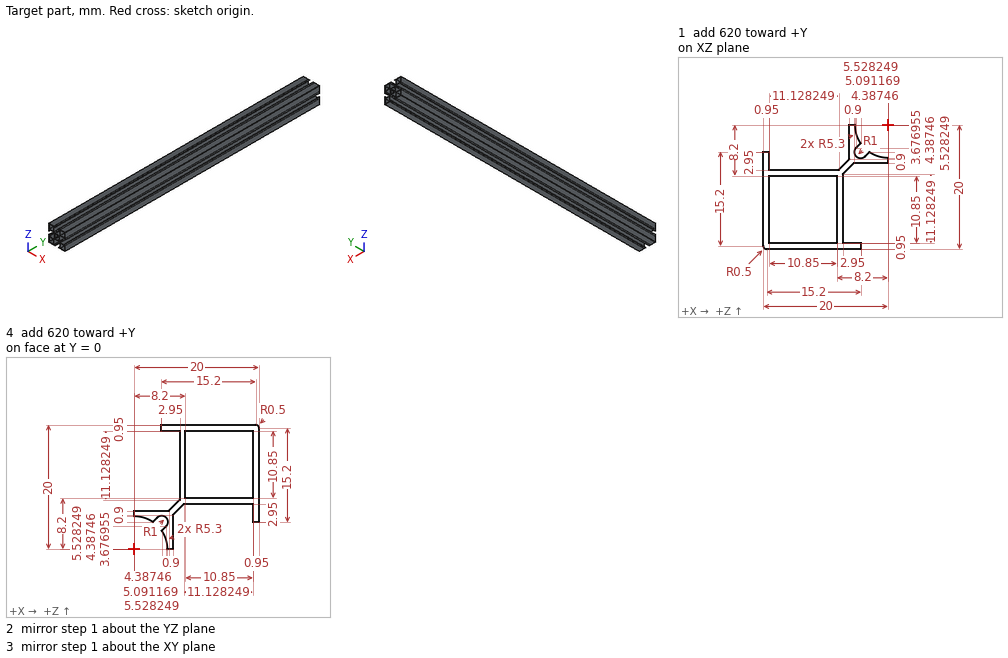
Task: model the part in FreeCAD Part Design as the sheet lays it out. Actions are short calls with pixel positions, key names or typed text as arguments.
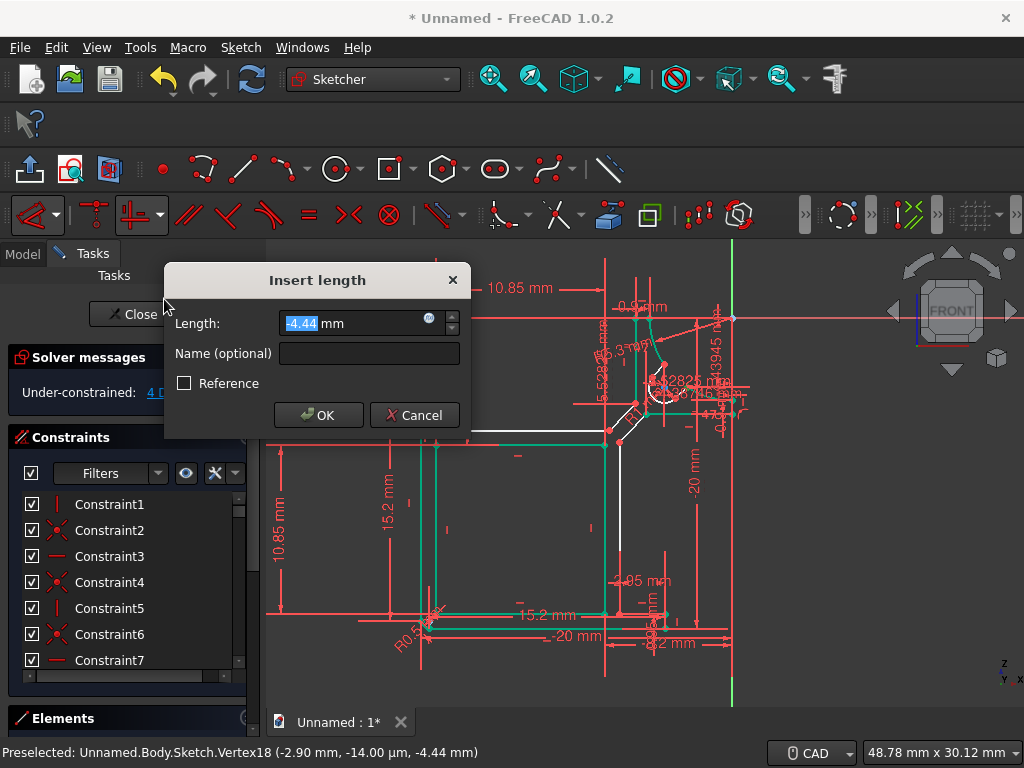
text(-4.38746)
key(Return)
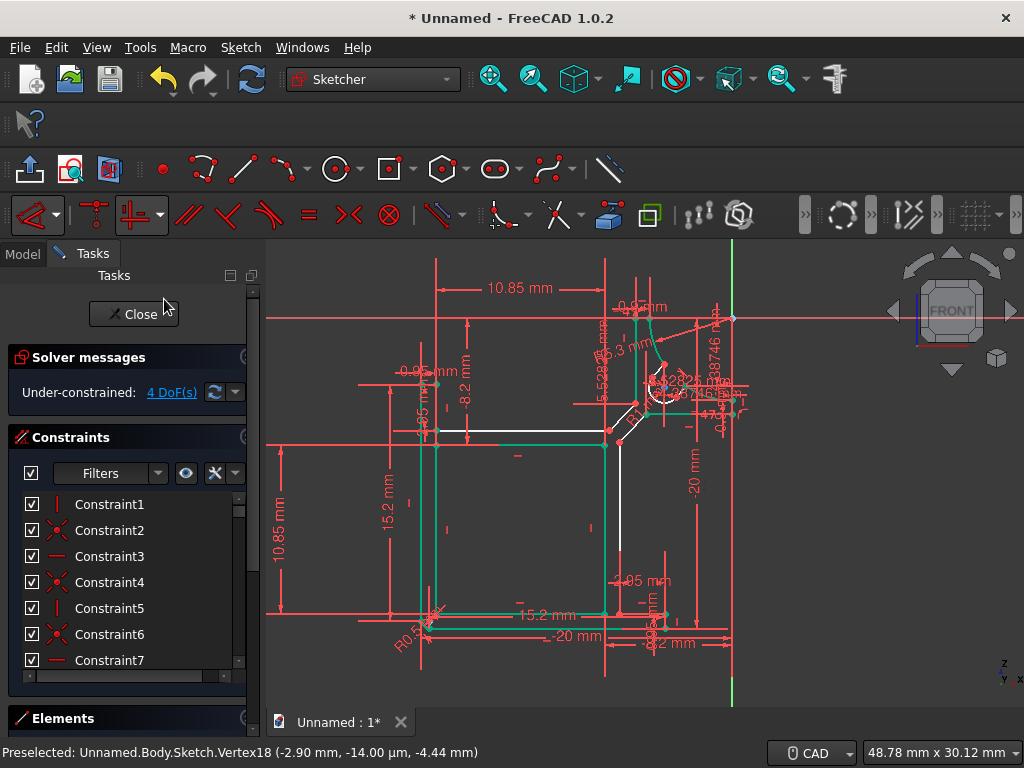
click(488, 431)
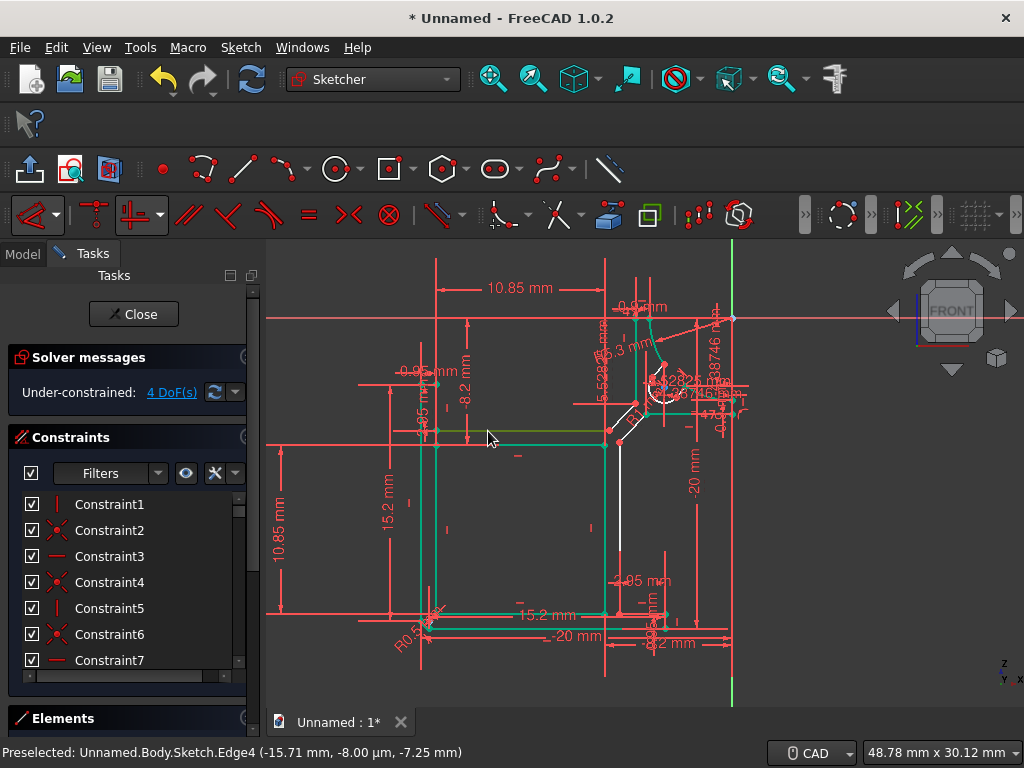
click(58, 216)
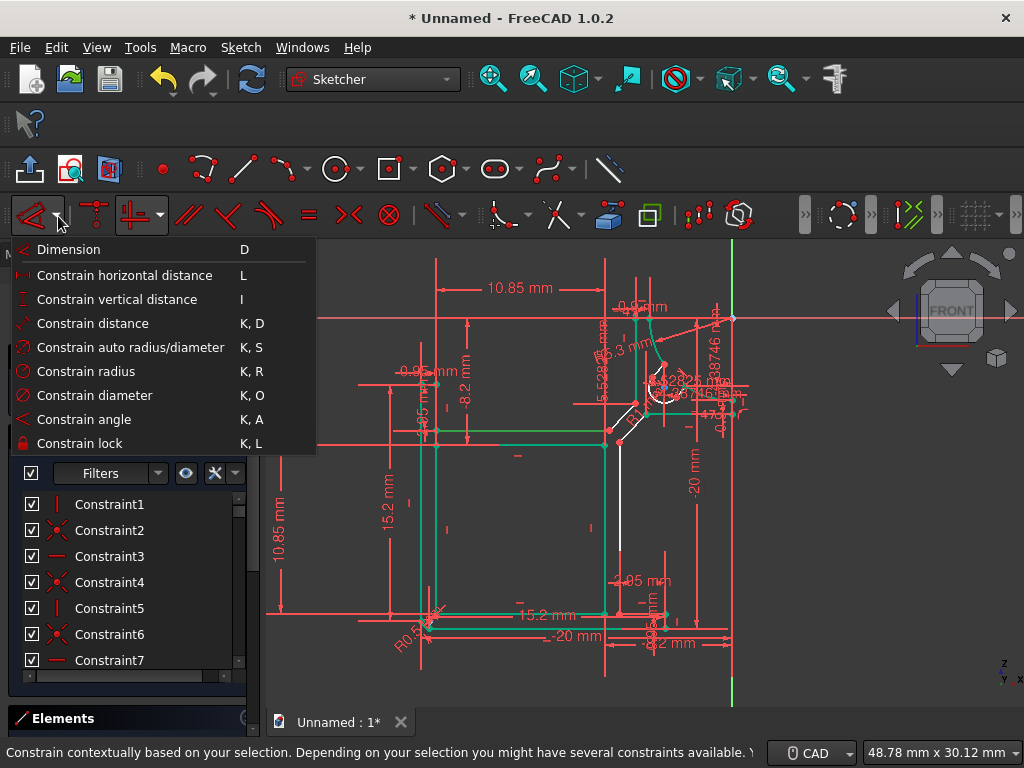
click(164, 275)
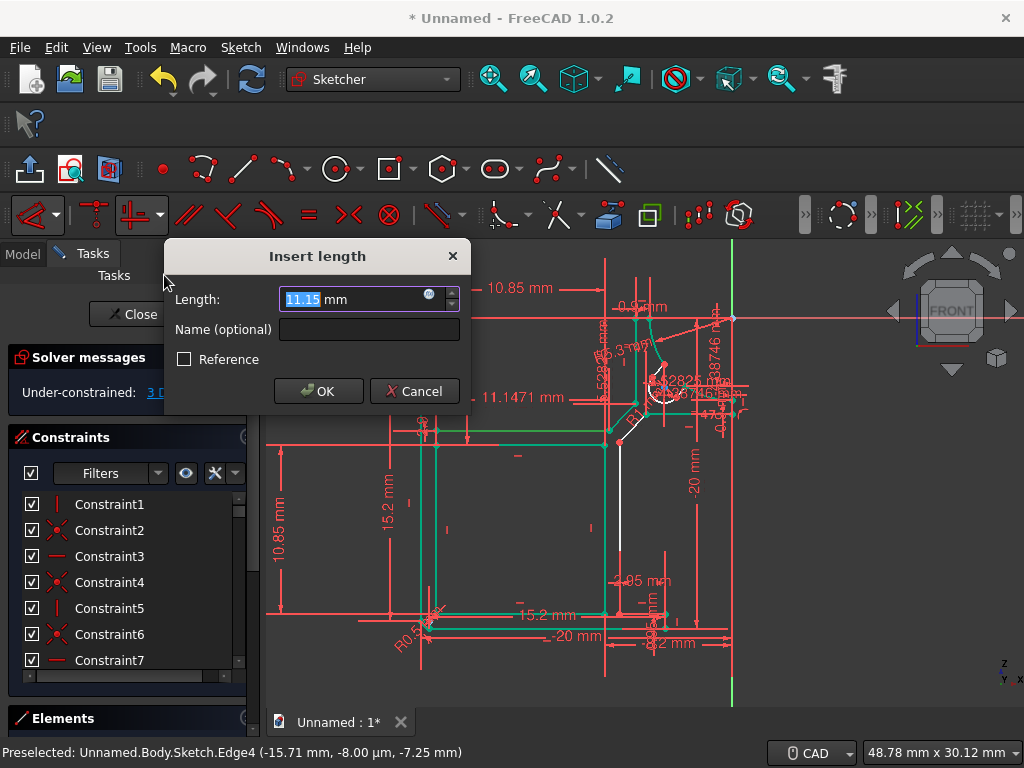
text(11.128249)
key(Return)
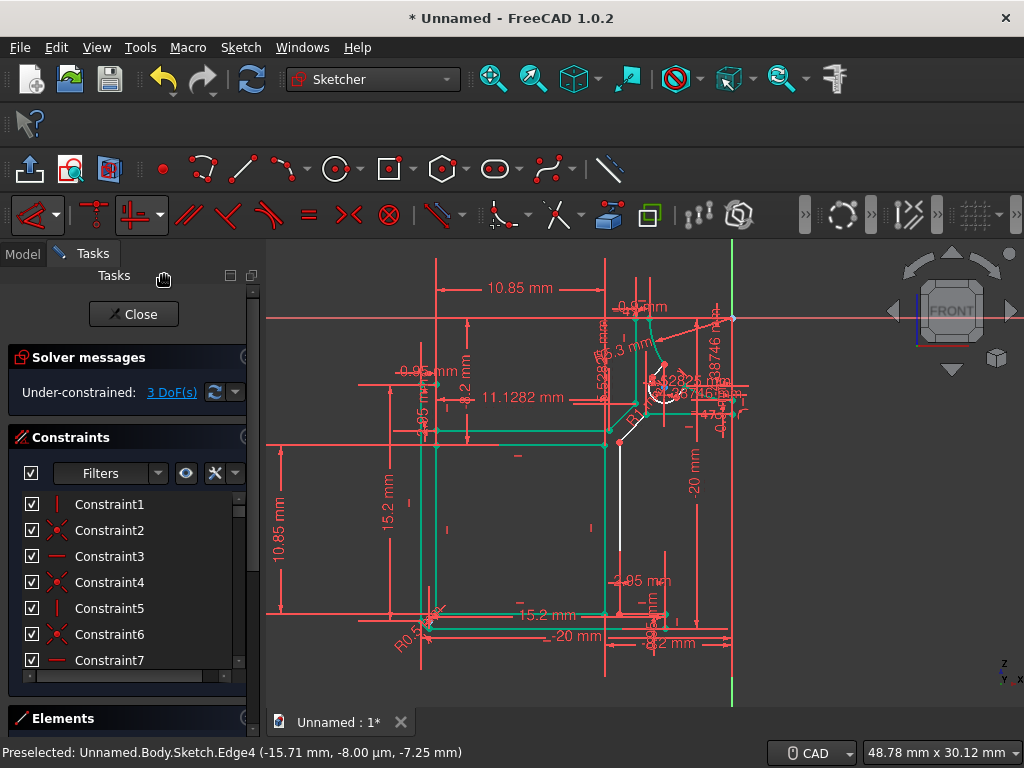
click(620, 494)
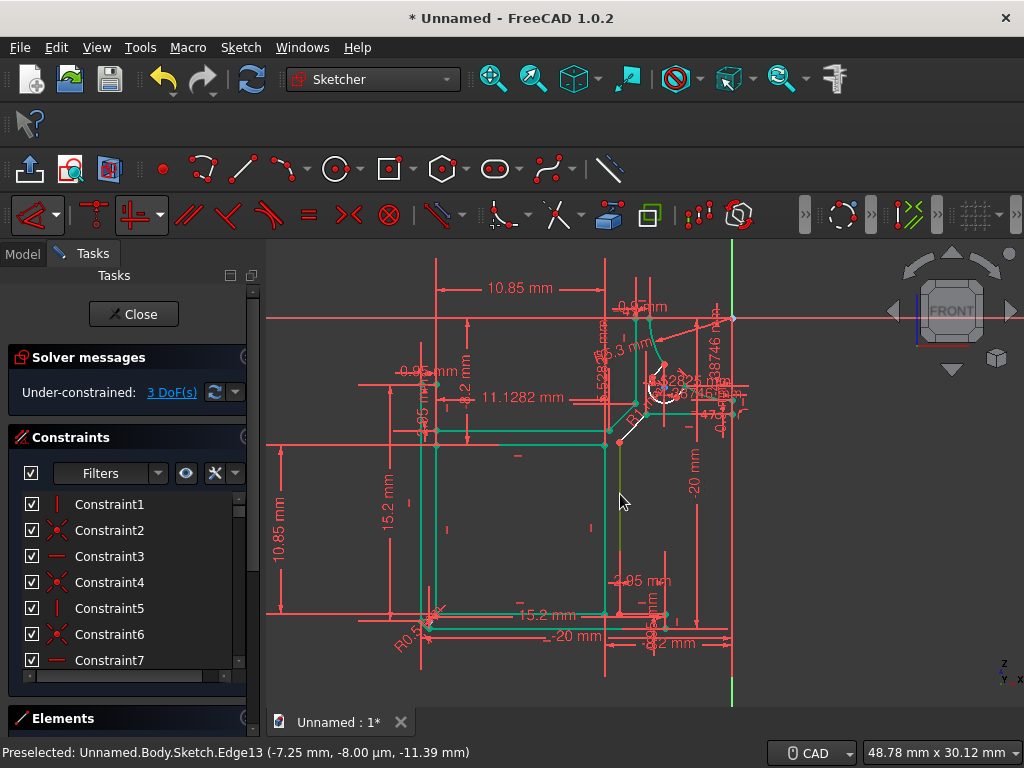
key(i)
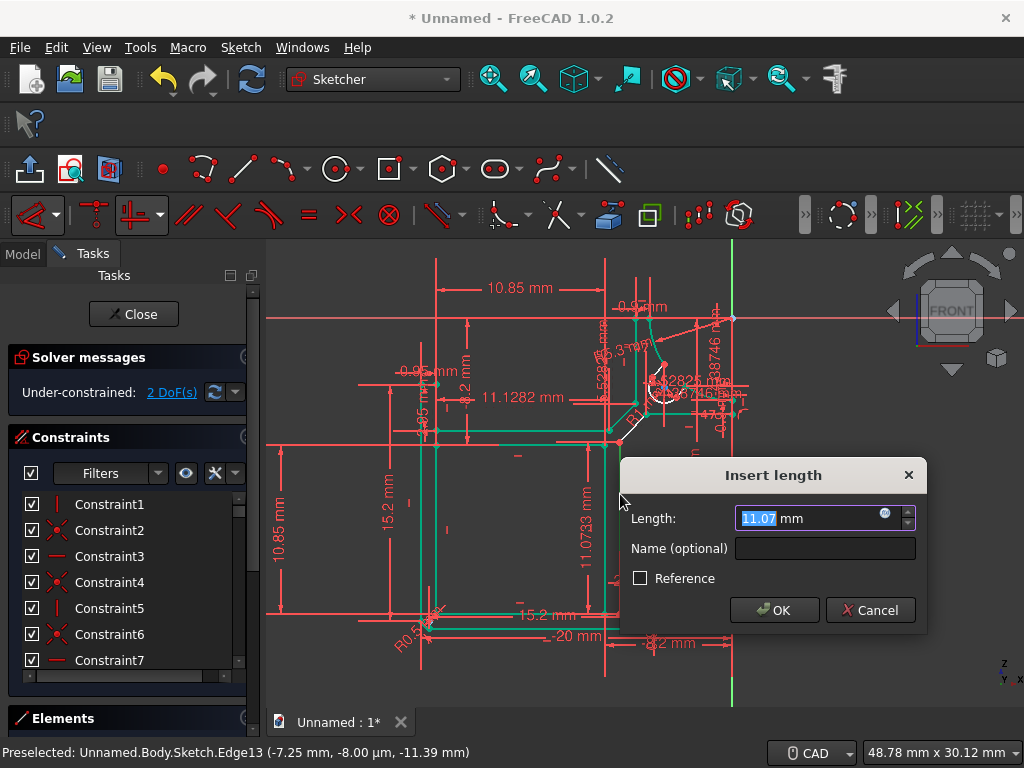
text(11.128249)
key(Return)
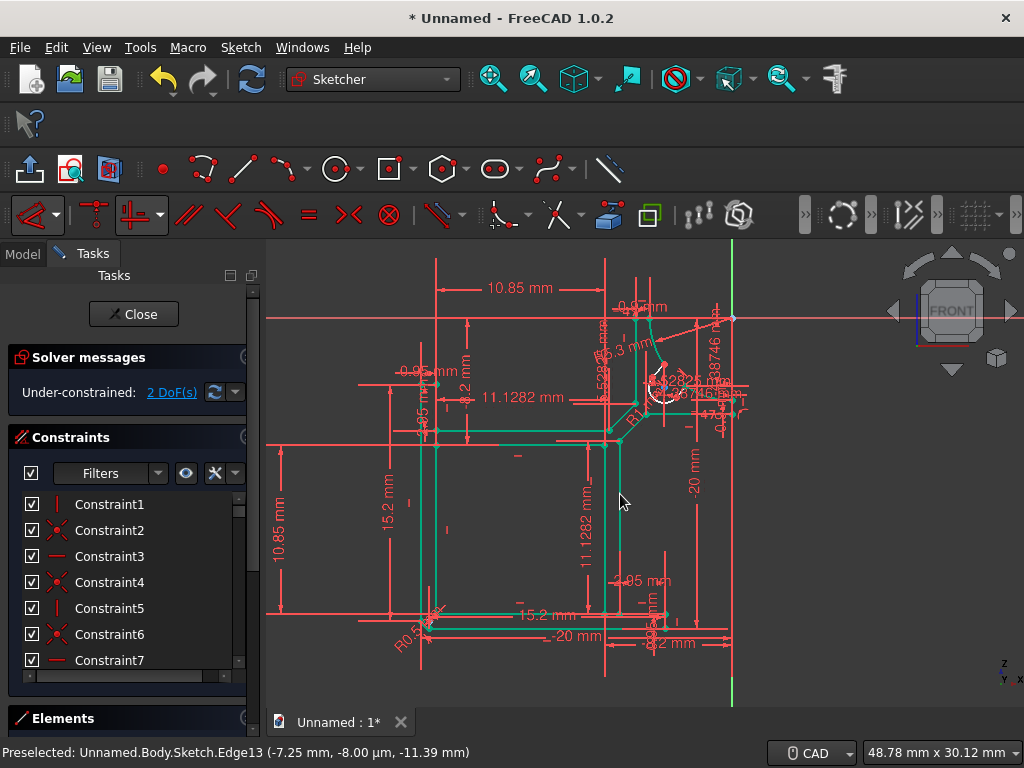
click(653, 377)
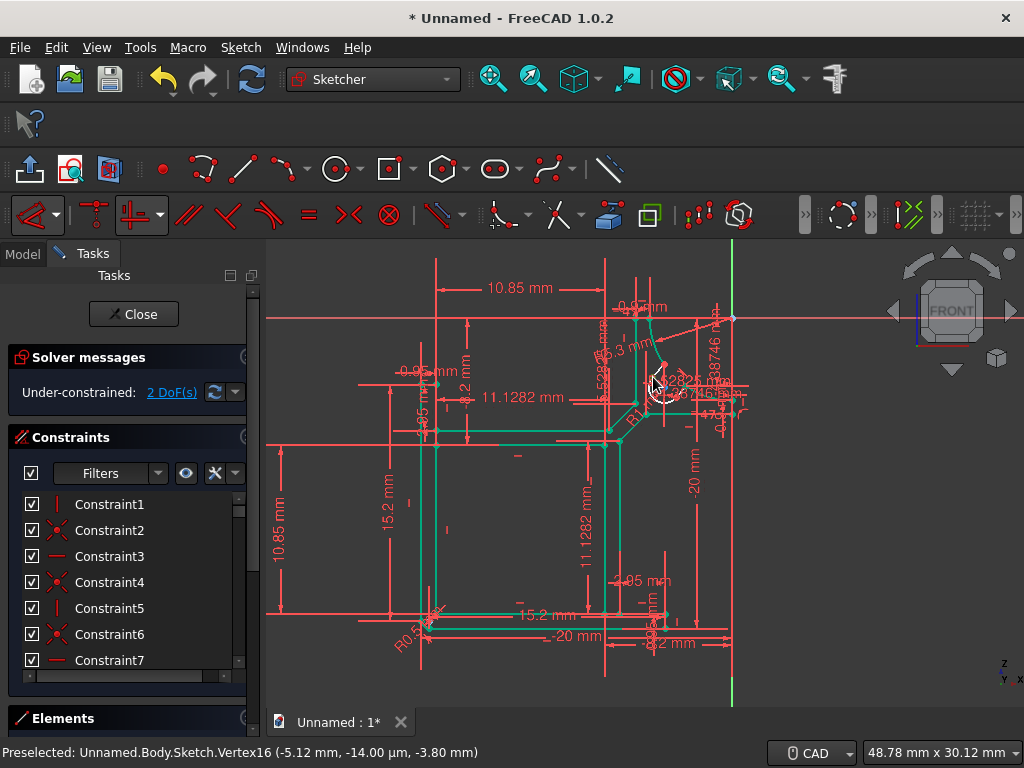
key(l)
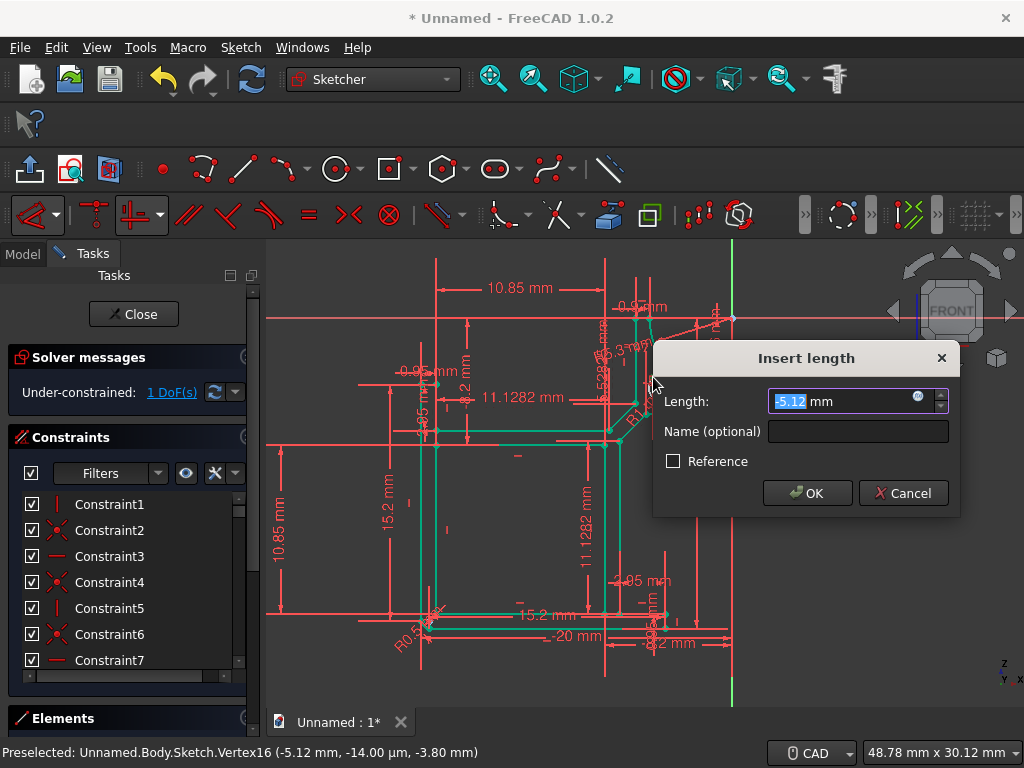
text(-5.091169)
key(Return)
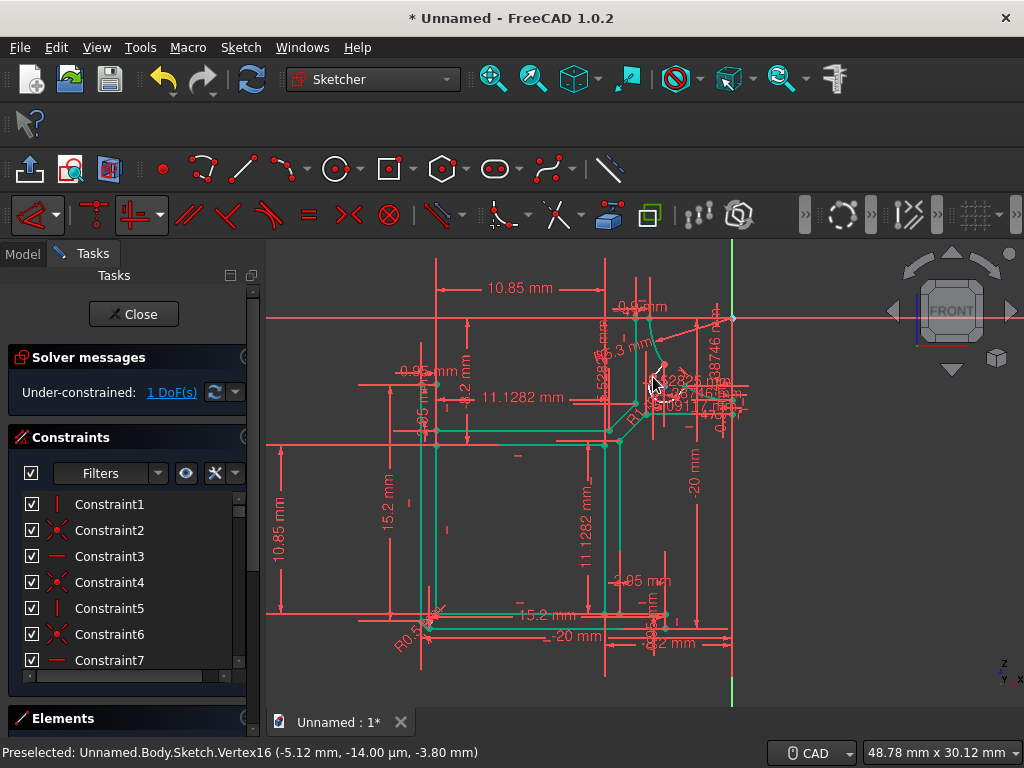
click(653, 377)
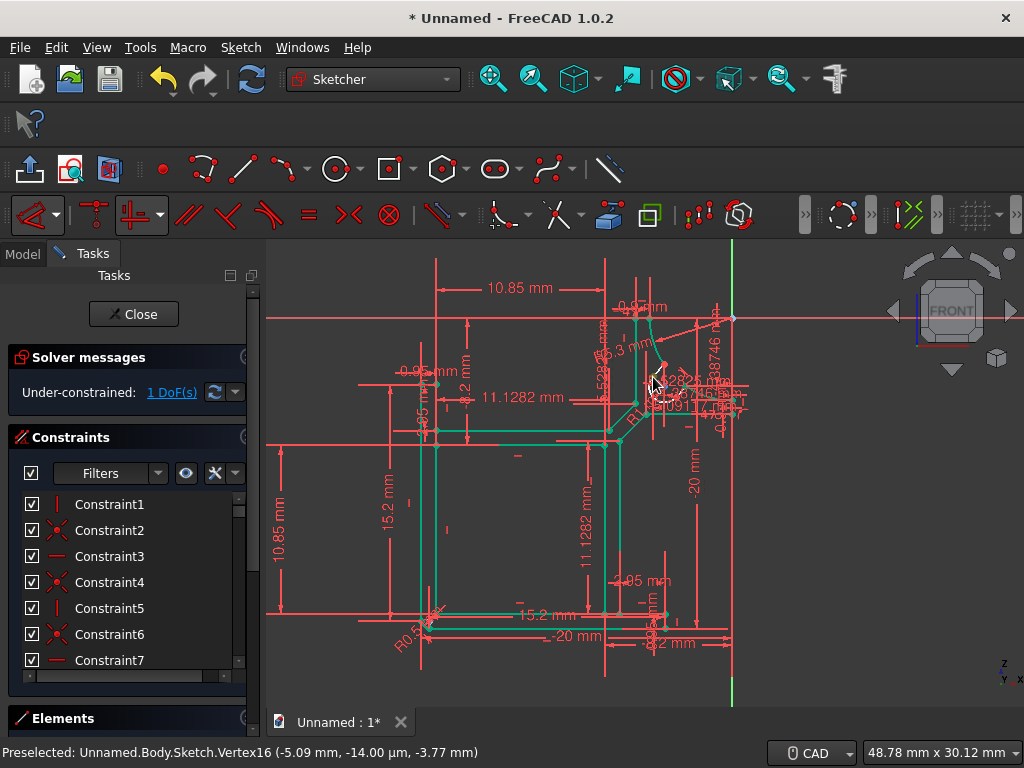
click(58, 216)